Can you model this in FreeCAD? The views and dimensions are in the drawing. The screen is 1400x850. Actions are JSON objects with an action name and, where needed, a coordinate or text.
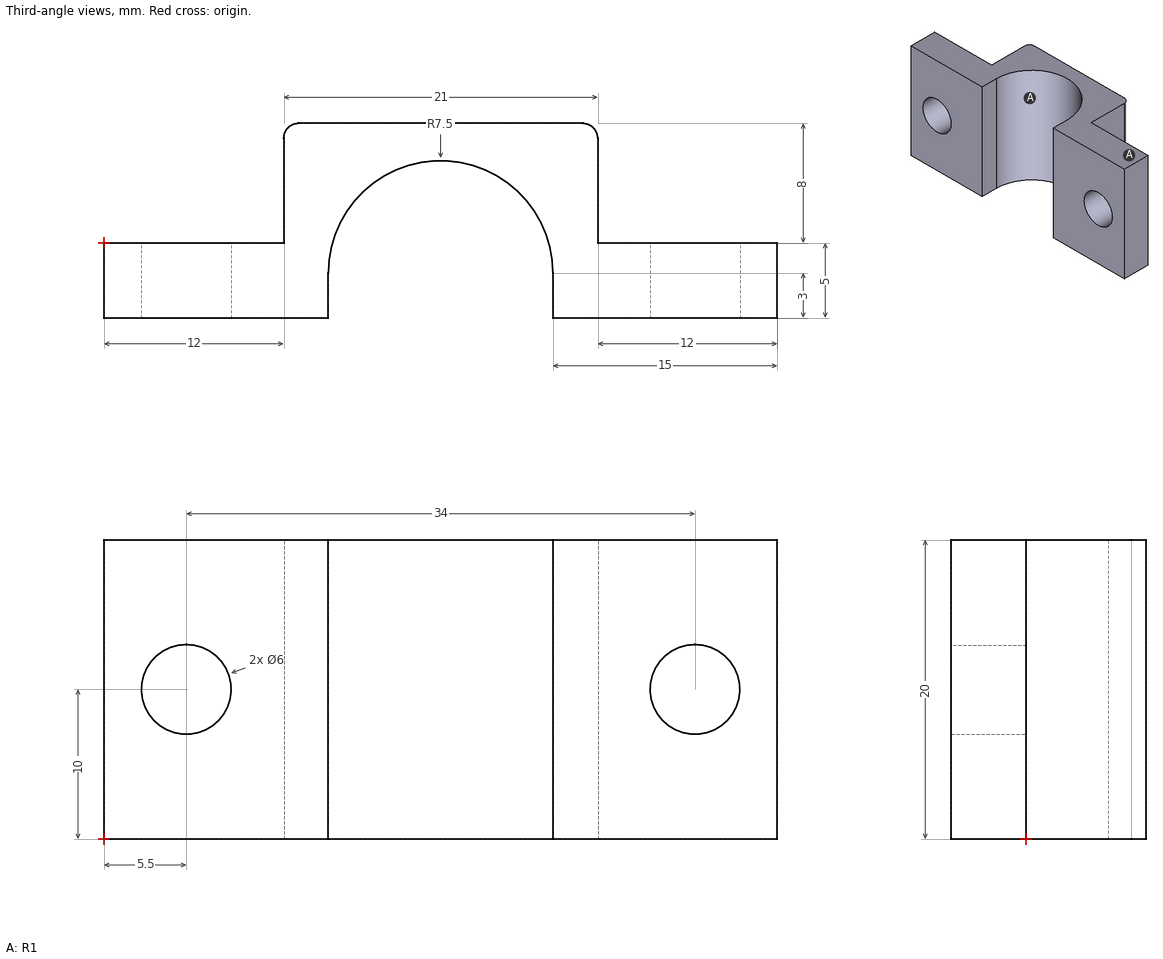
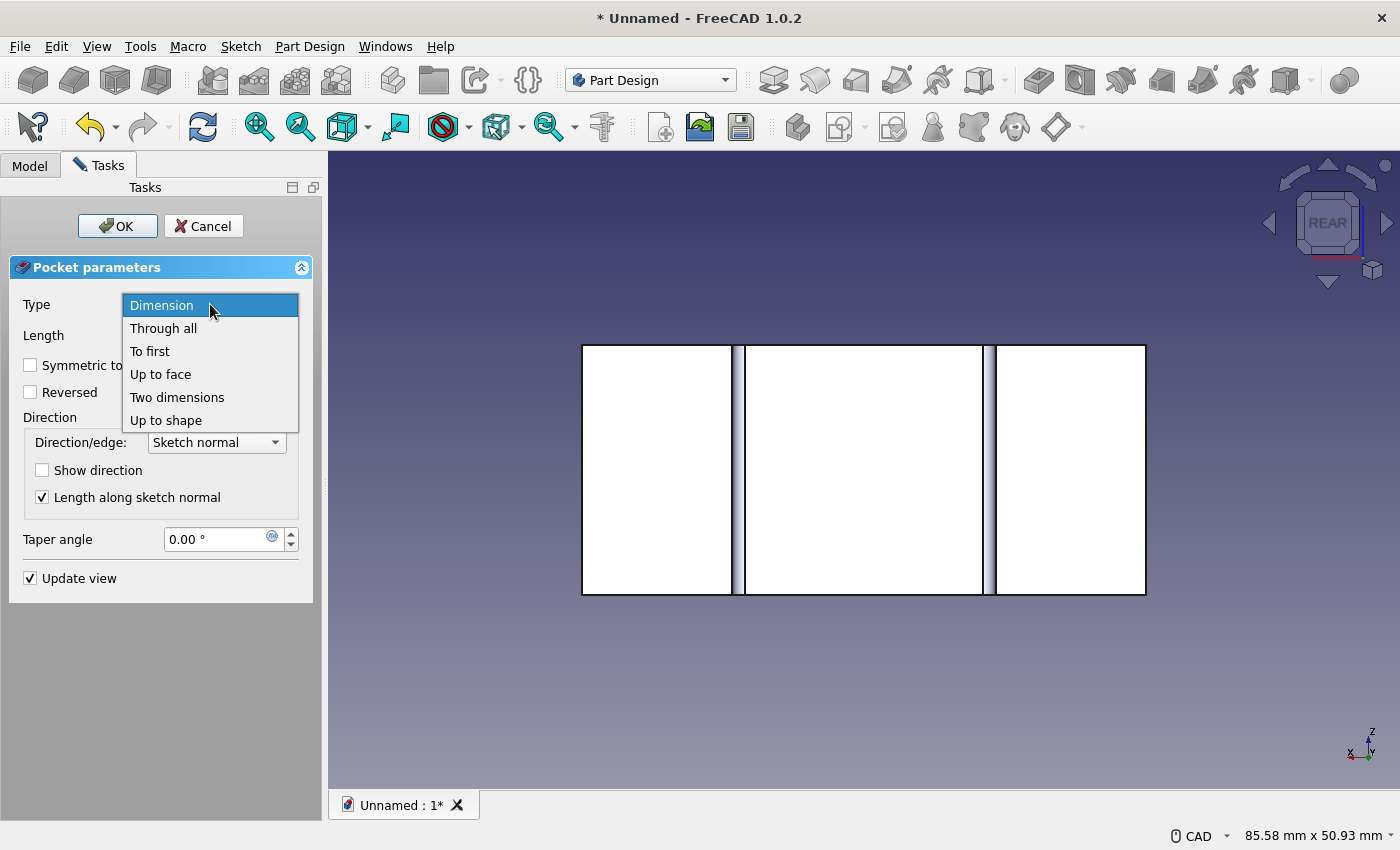
{"action": "left_click", "coordinate": [208, 328]}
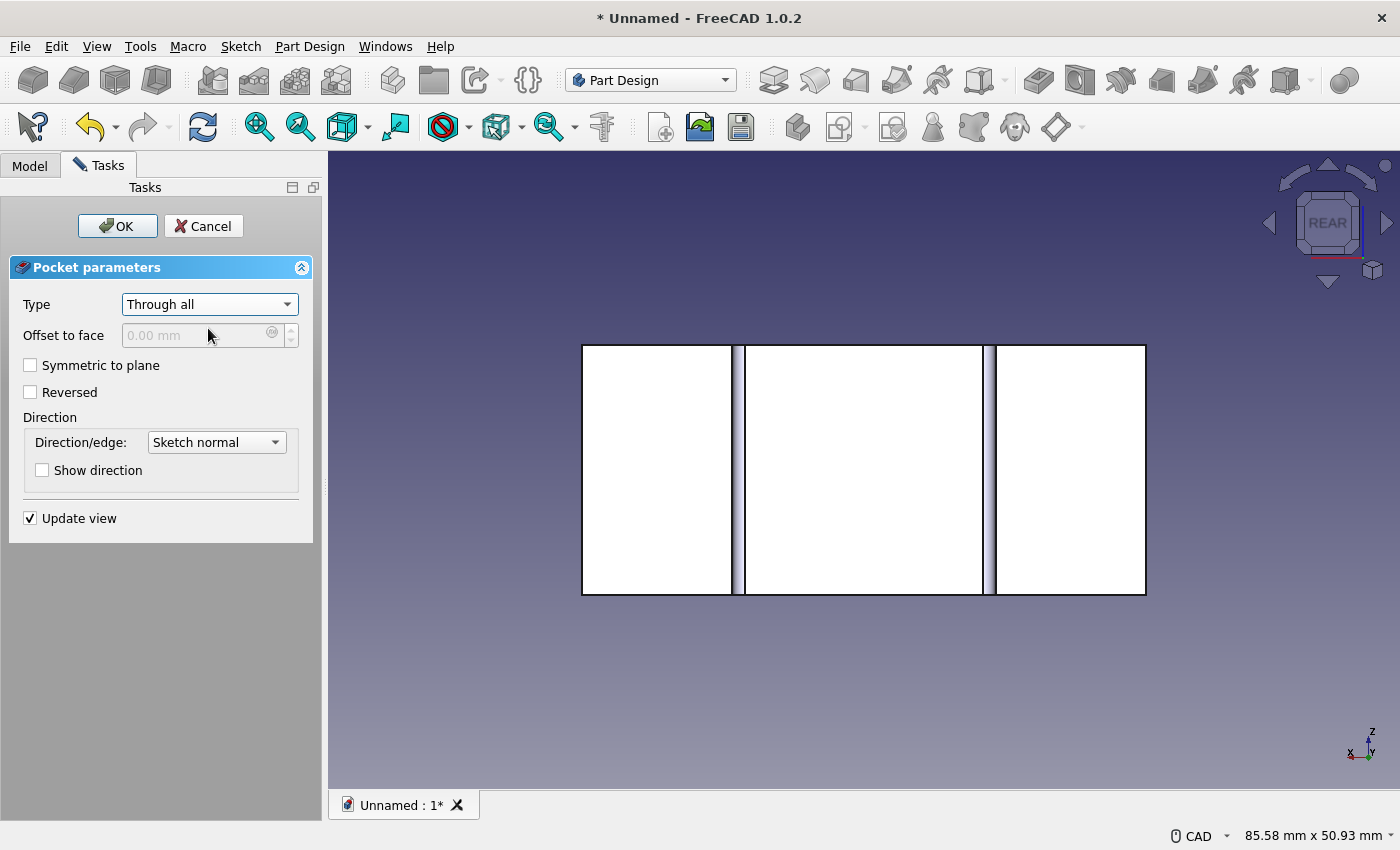
{"action": "left_click", "coordinate": [31, 392]}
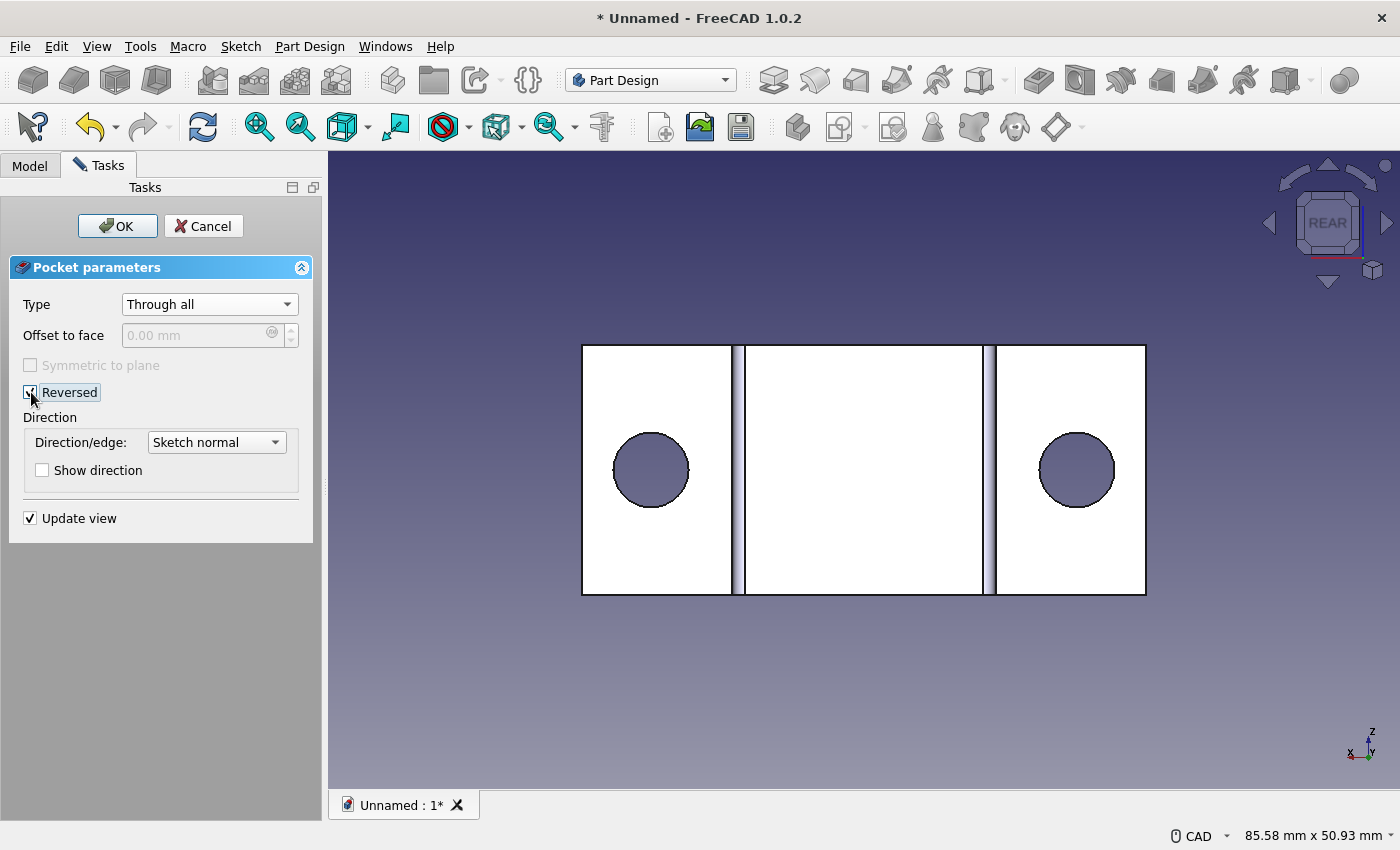
{"action": "left_click", "coordinate": [118, 226]}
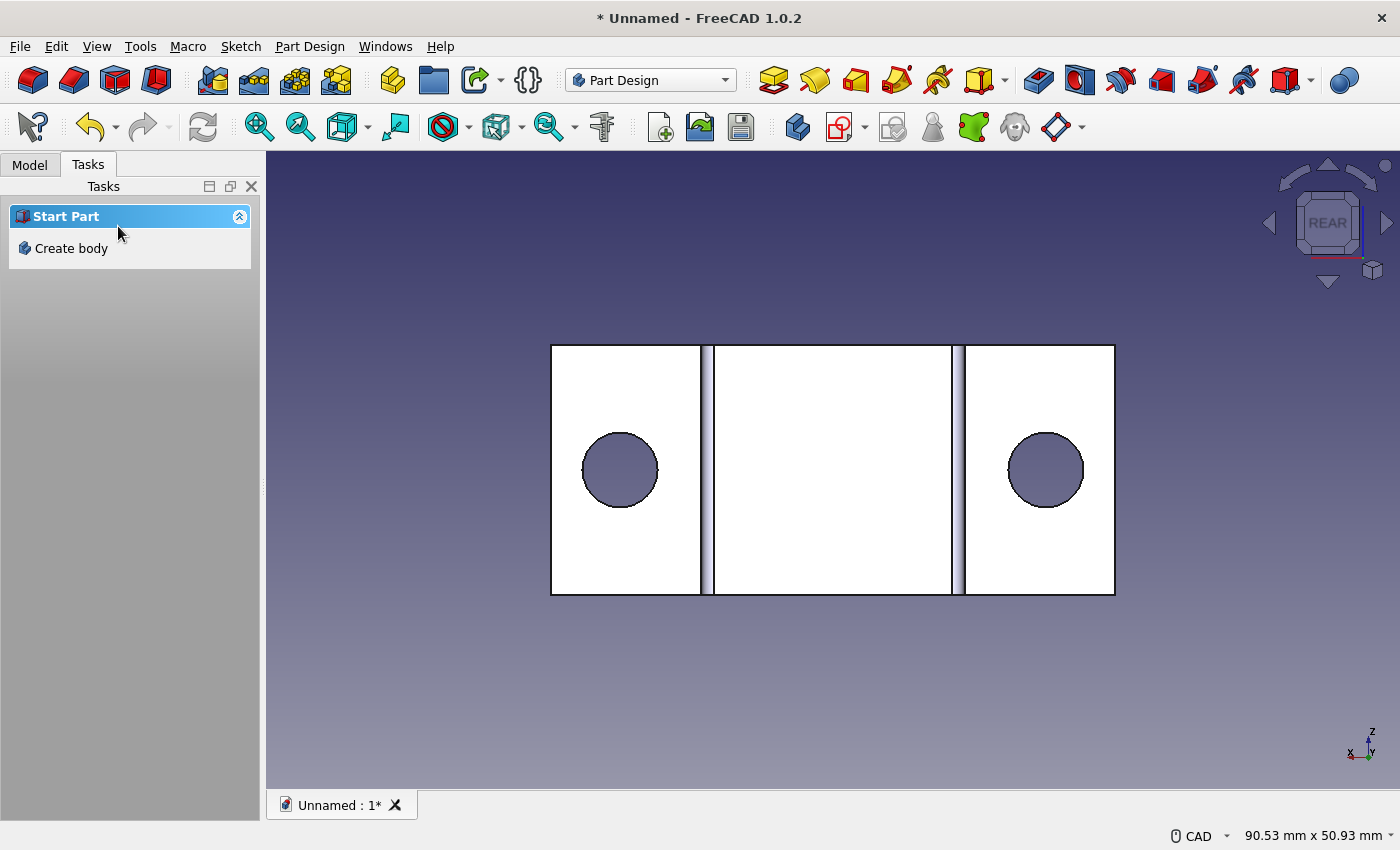
{"action": "key", "text": "0"}